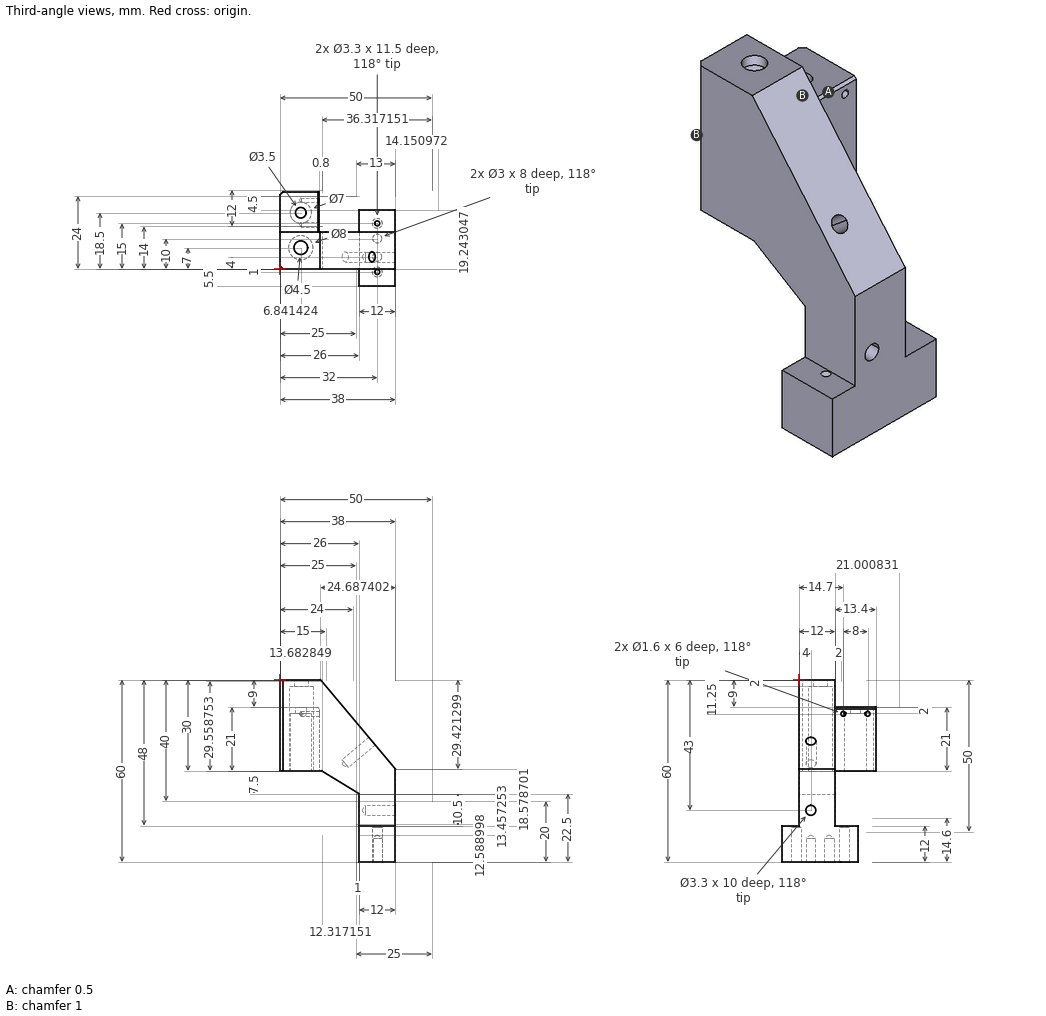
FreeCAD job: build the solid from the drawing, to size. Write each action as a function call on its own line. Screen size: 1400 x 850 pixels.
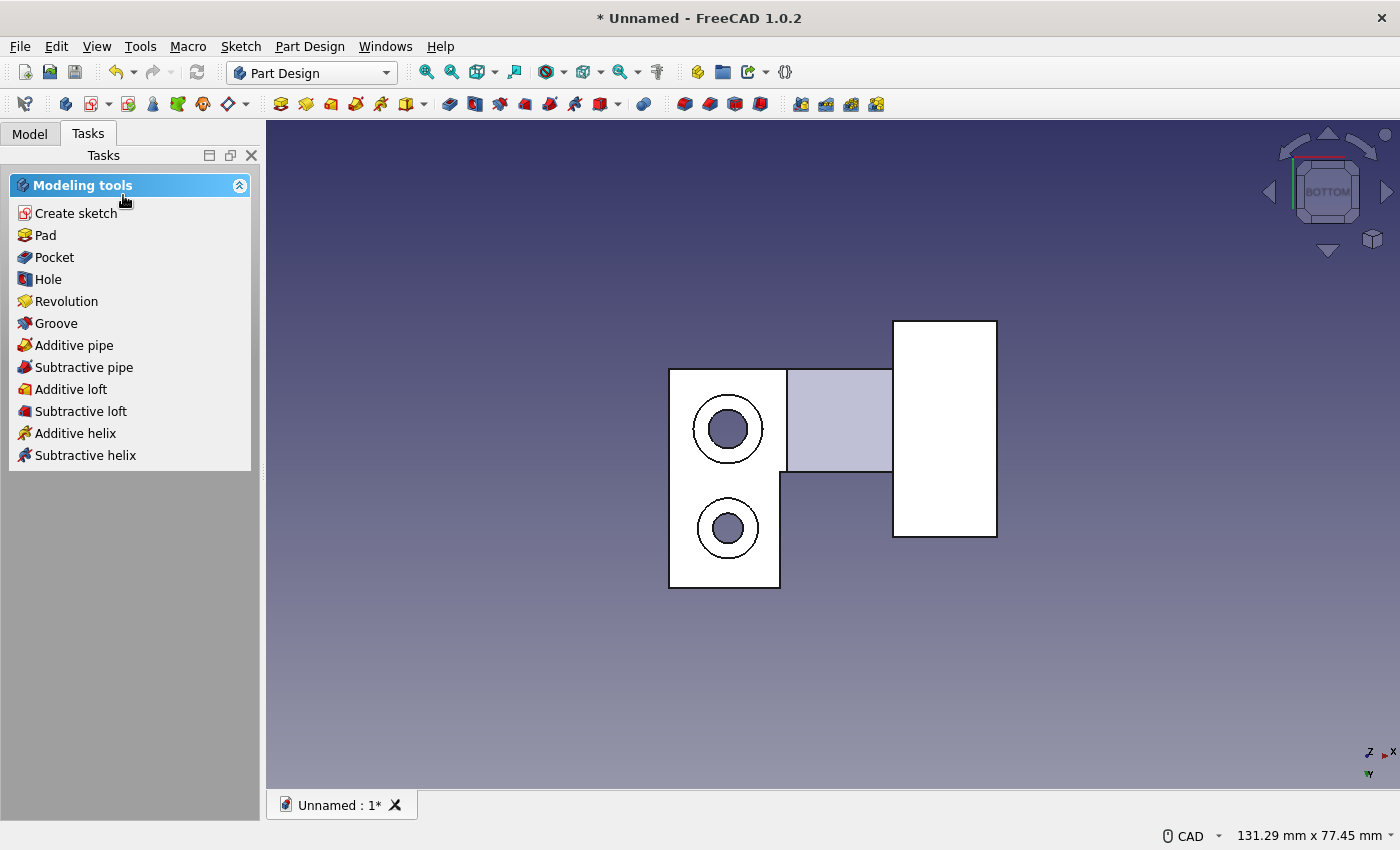
click(475, 104)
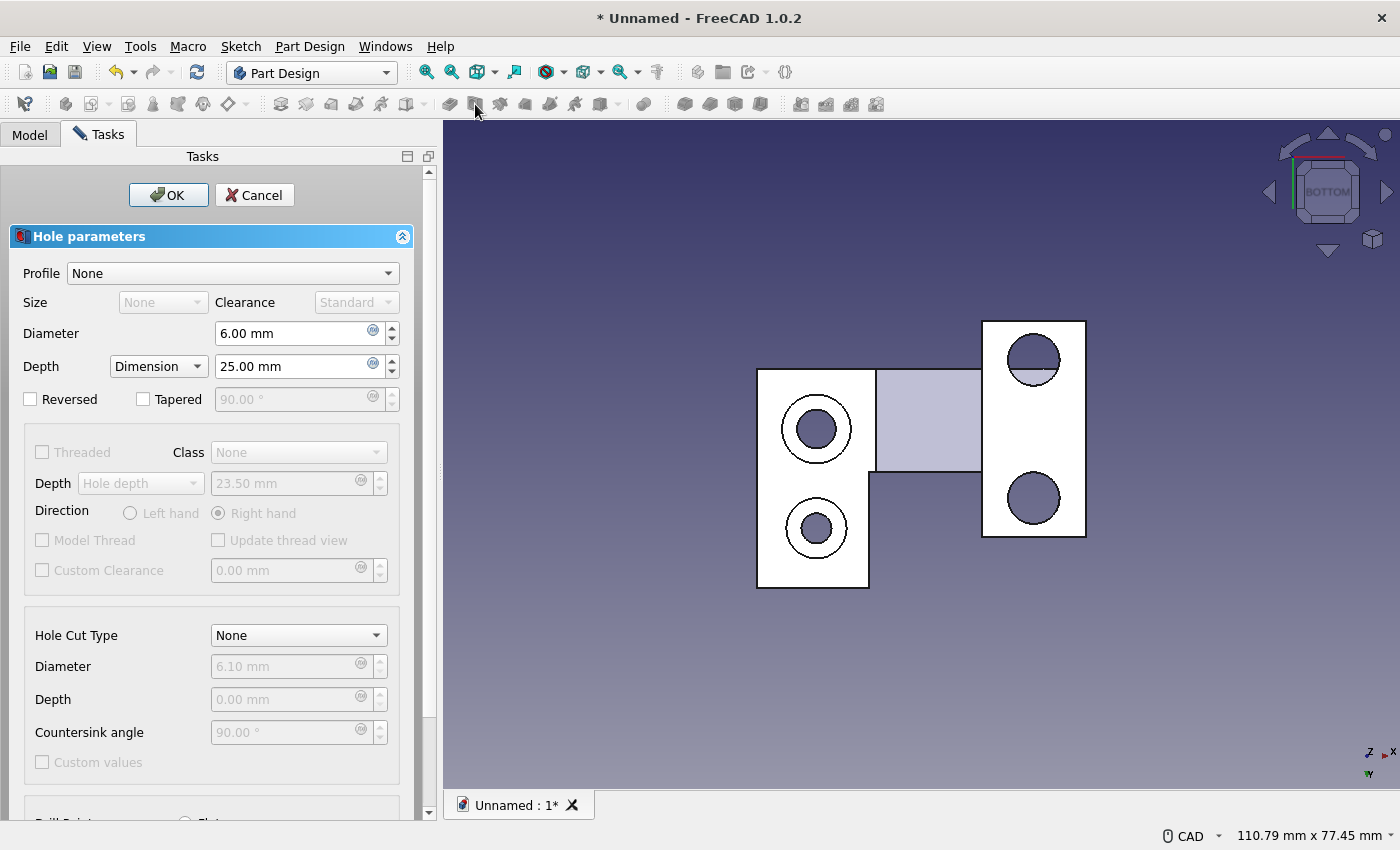
triple_click(300, 334)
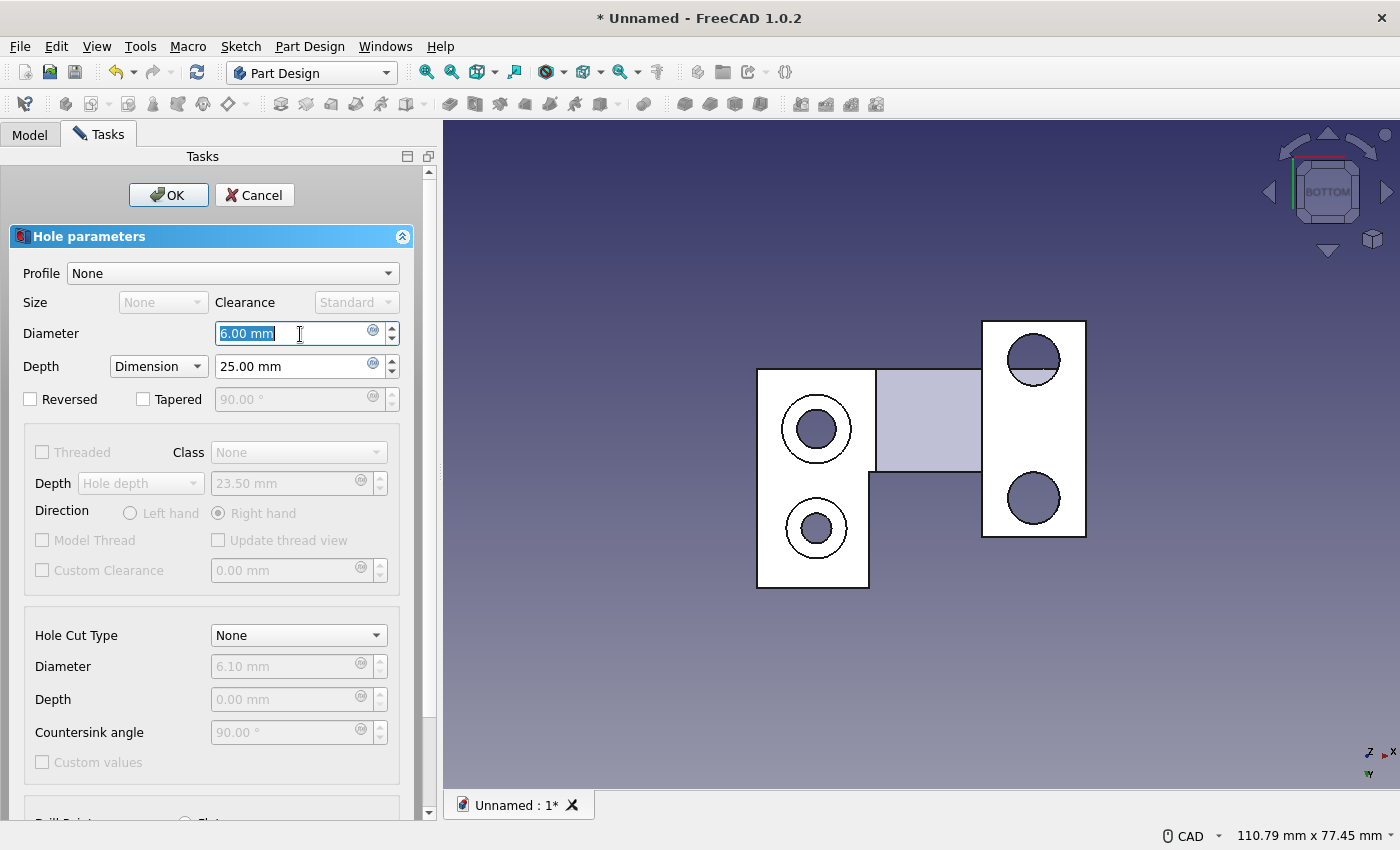
text(3.3)
key(Tab)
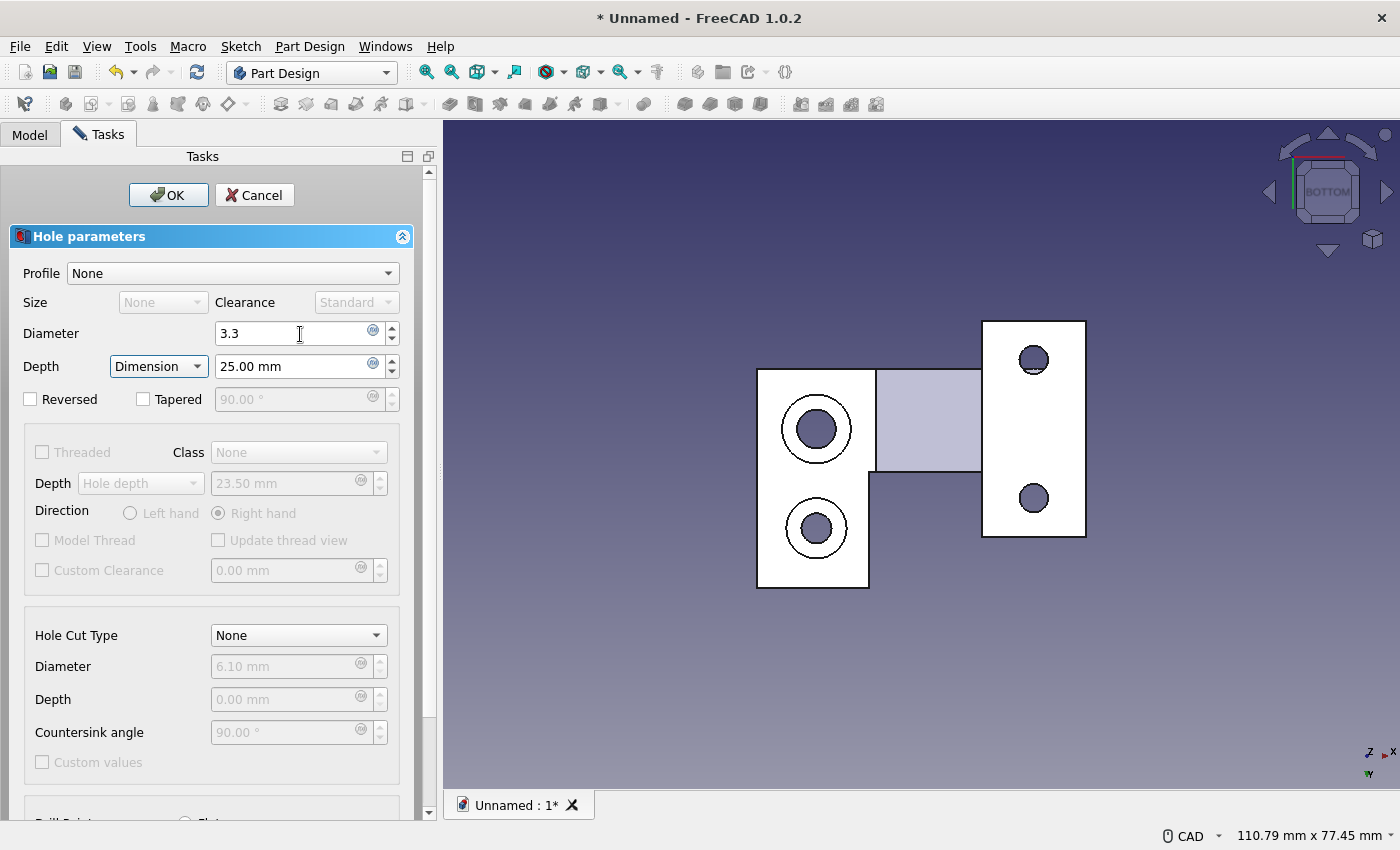
triple_click(300, 366)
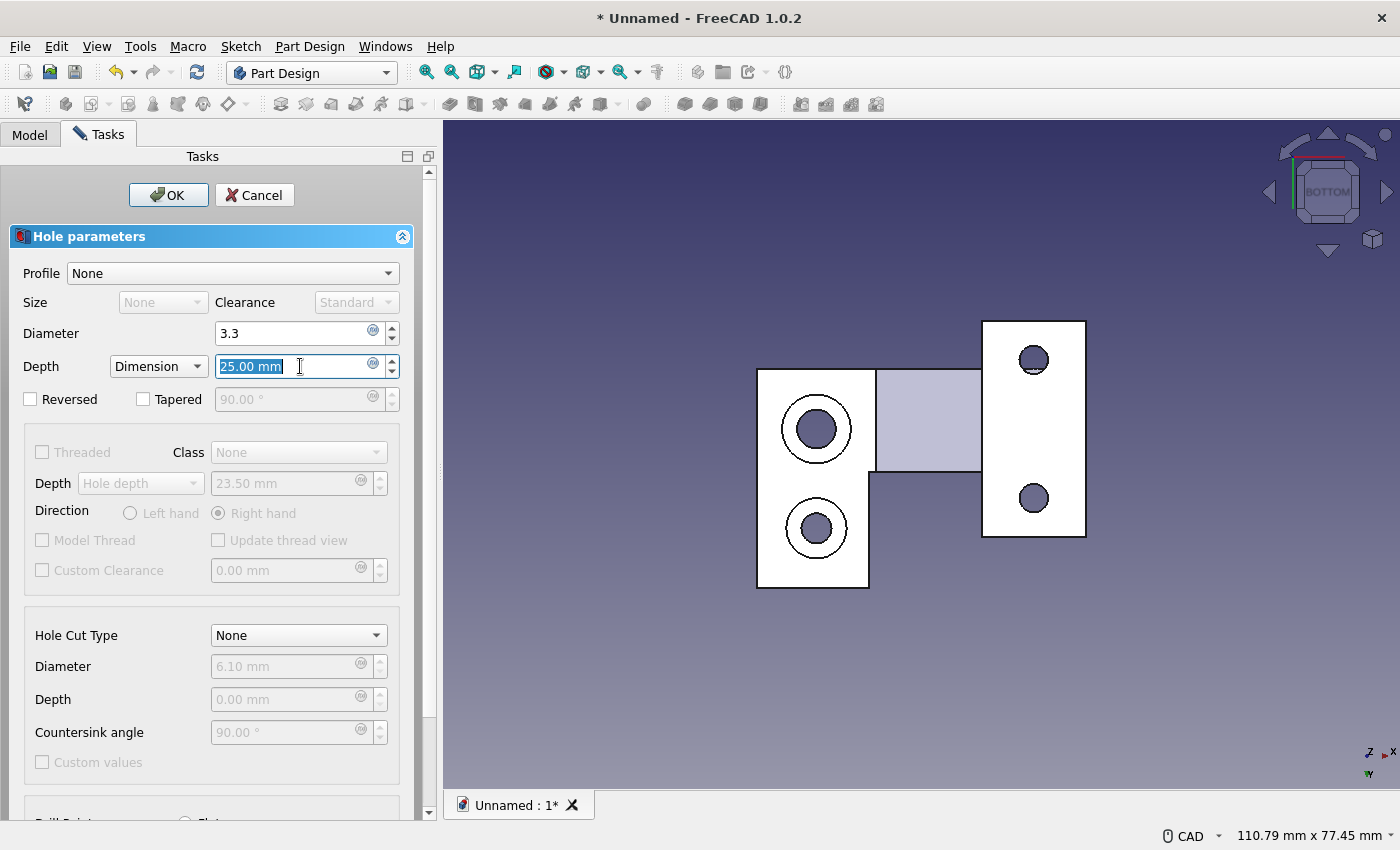
text(11.5)
key(Tab)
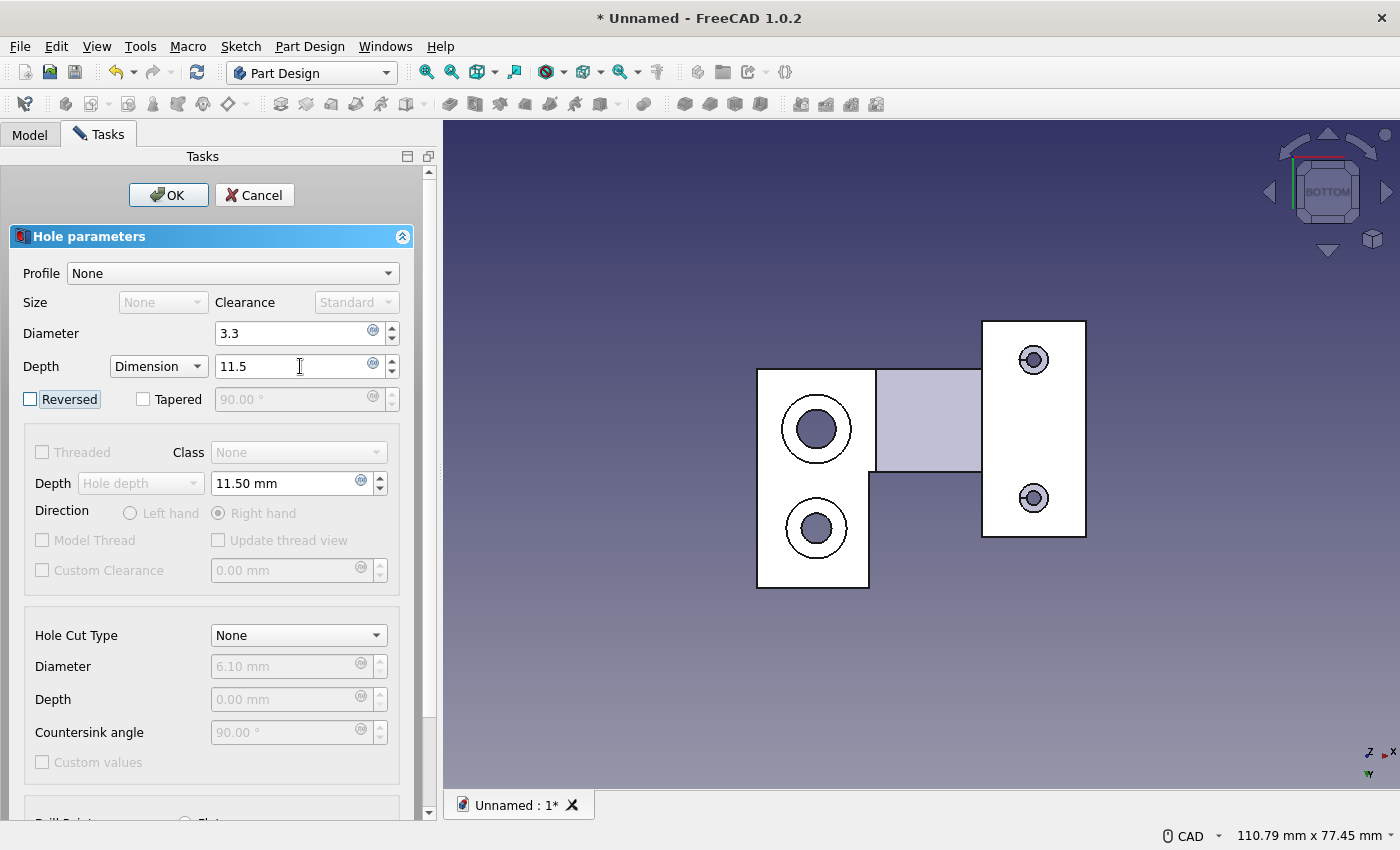
click(169, 195)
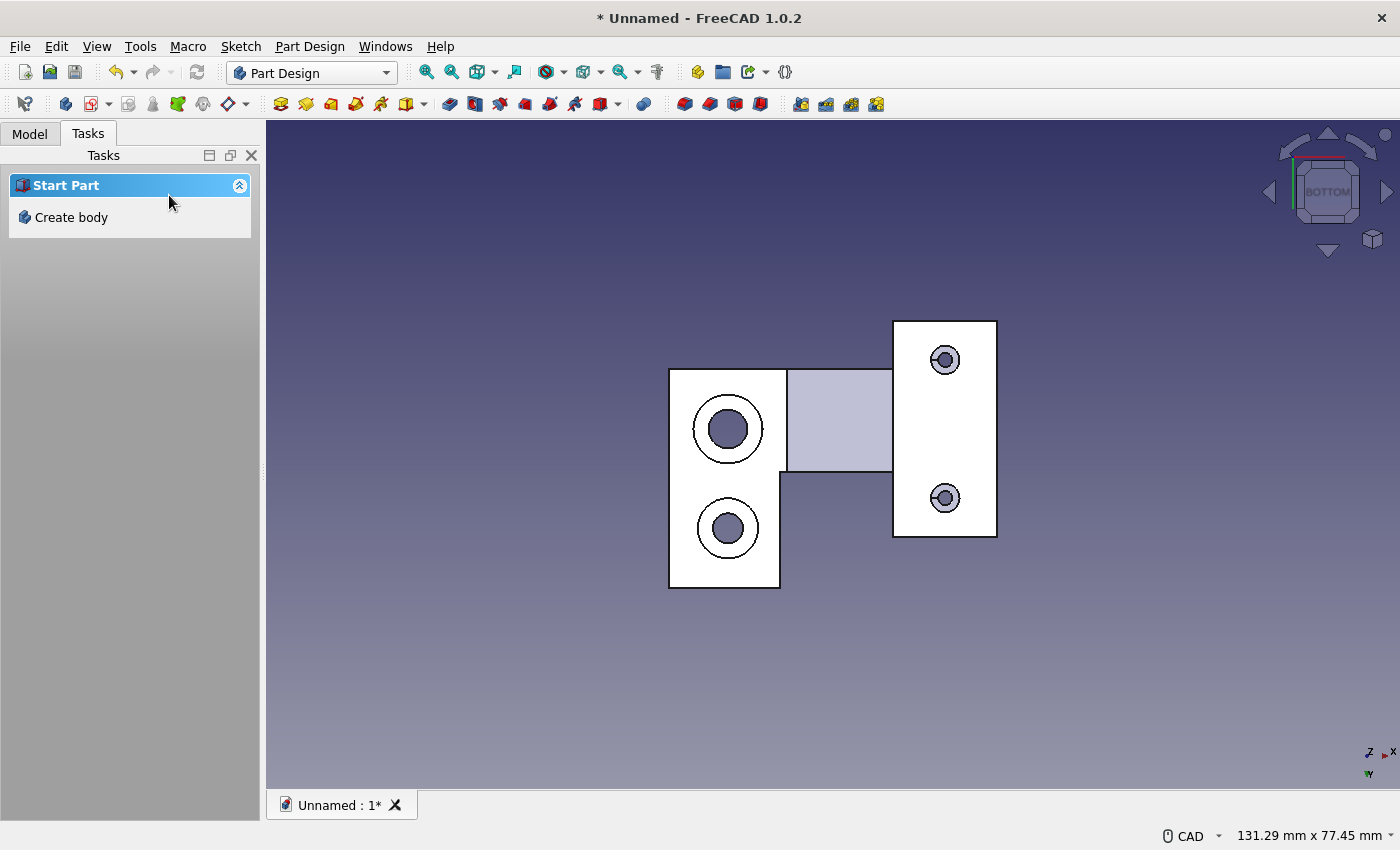
click(427, 72)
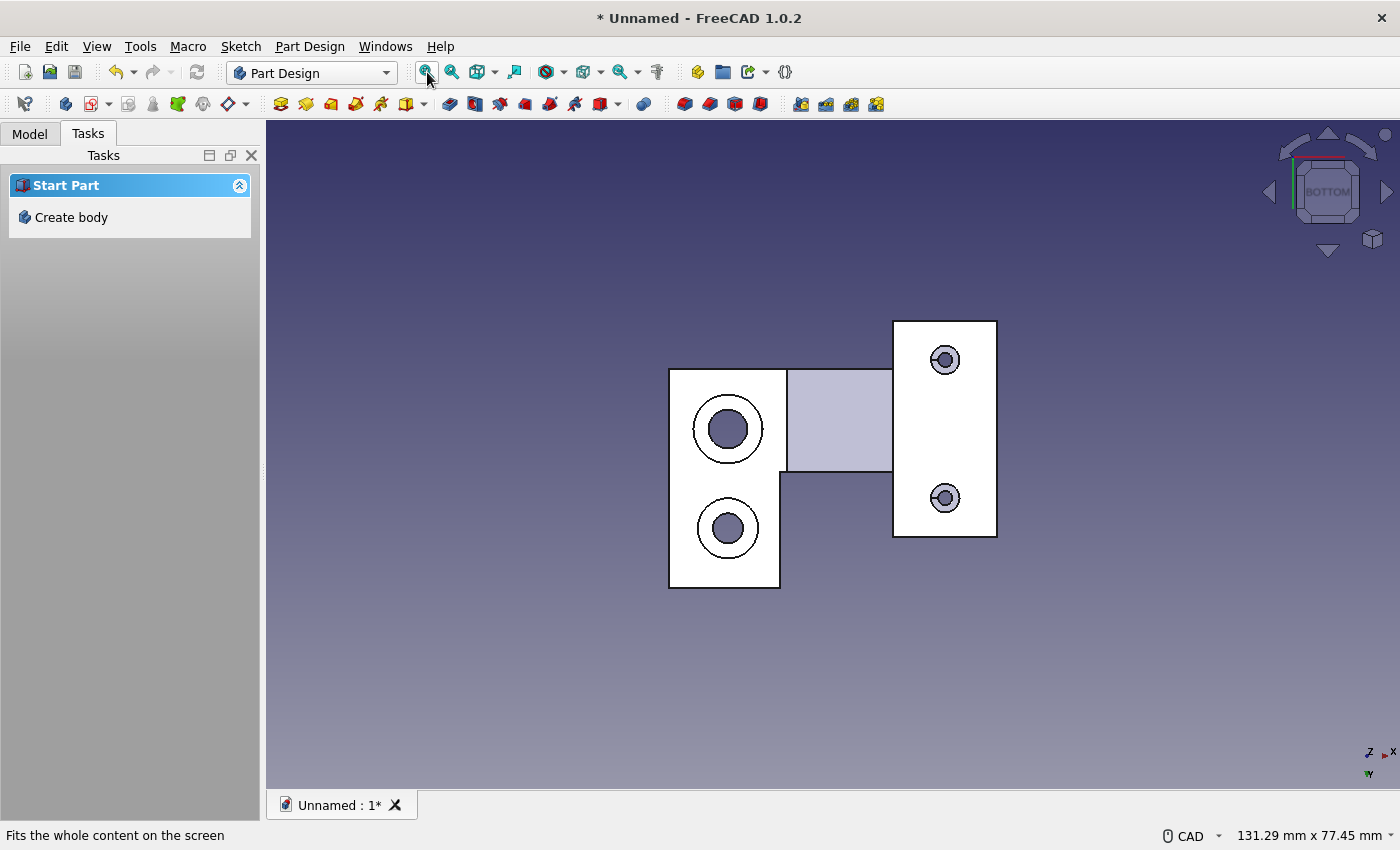
key(0)